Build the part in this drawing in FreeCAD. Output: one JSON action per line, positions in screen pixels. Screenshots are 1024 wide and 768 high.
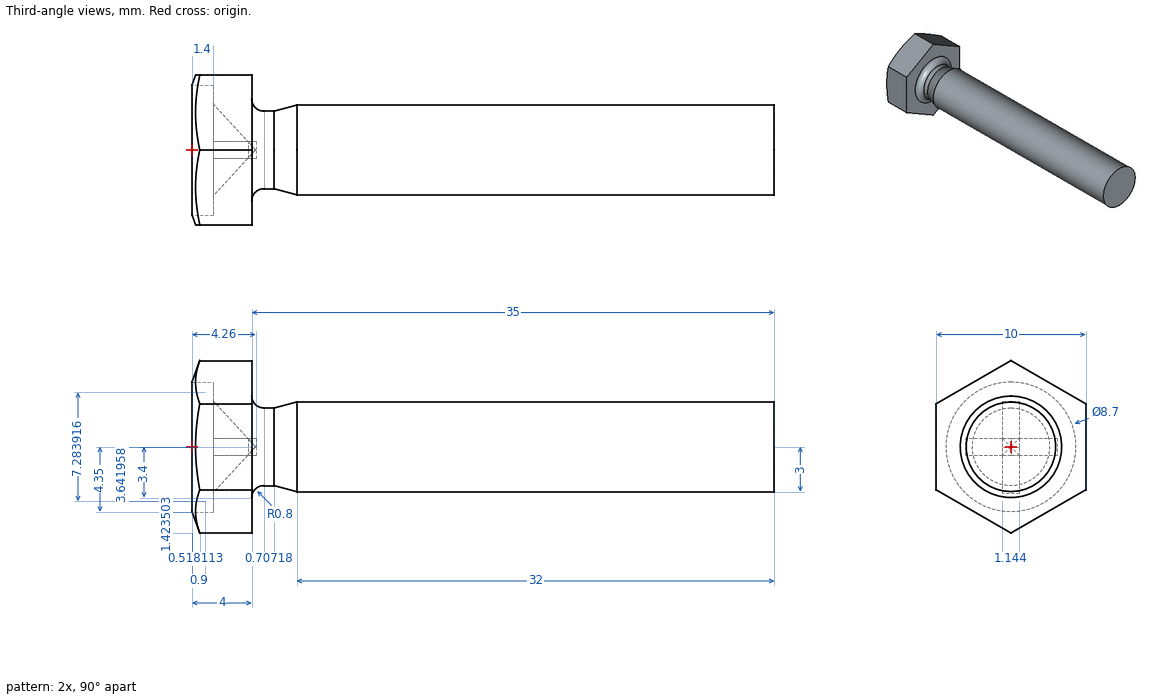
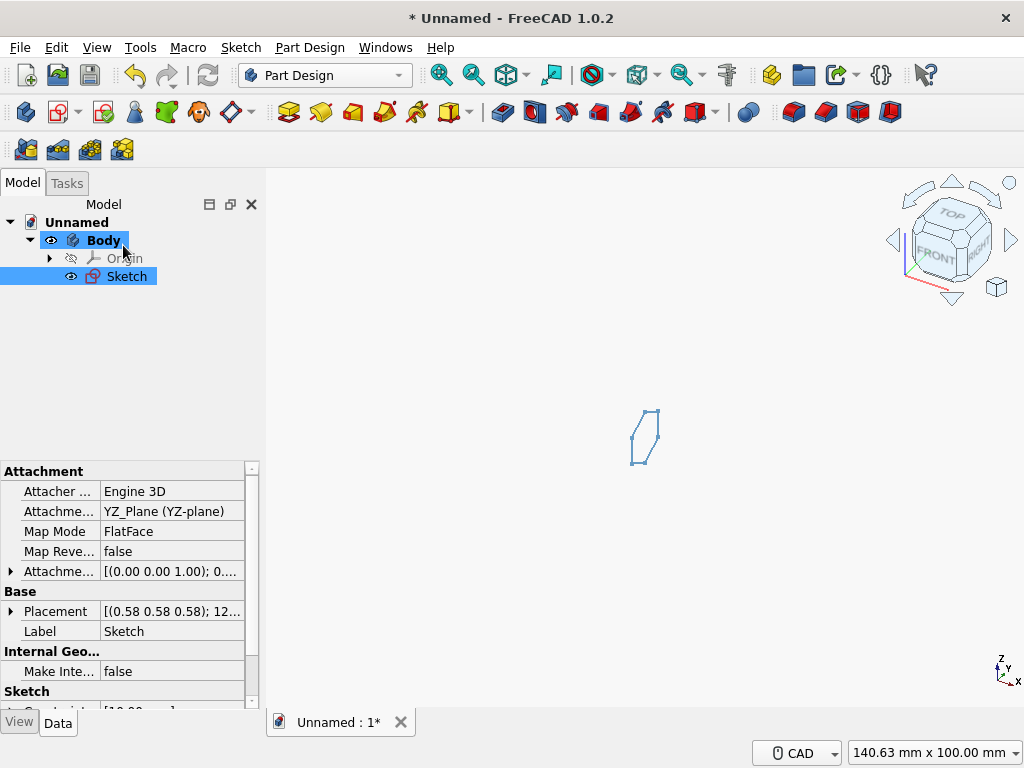
{"action": "left_click", "coordinate": [290, 112]}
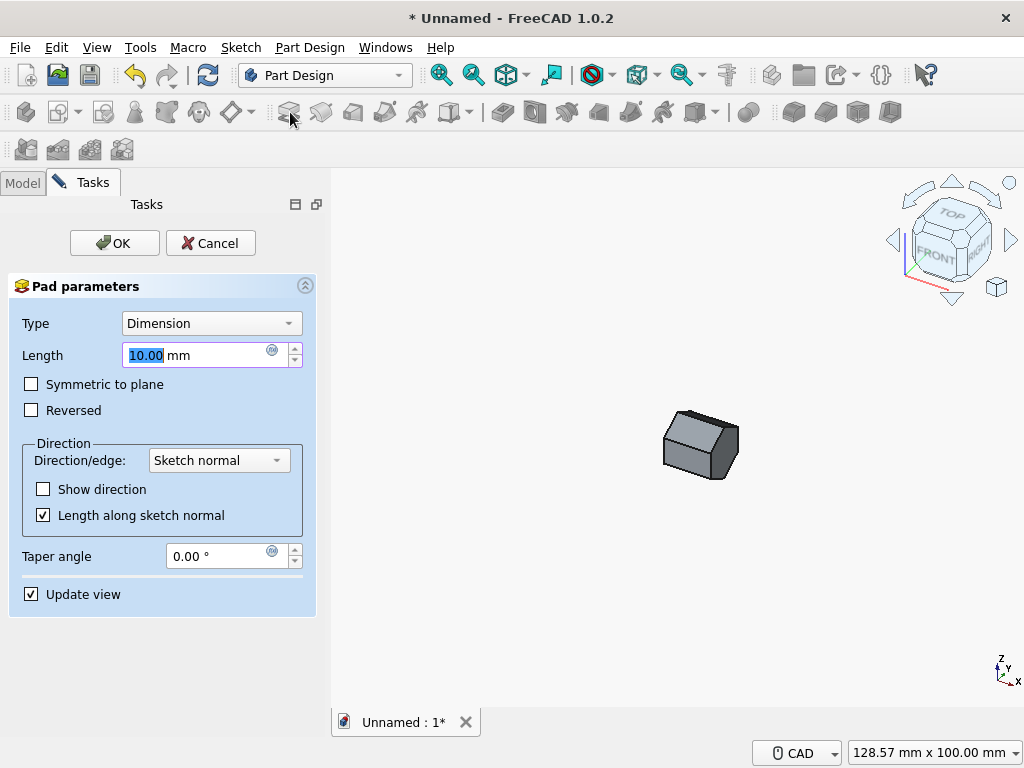
{"action": "type", "text": "4"}
{"action": "key", "text": "Tab"}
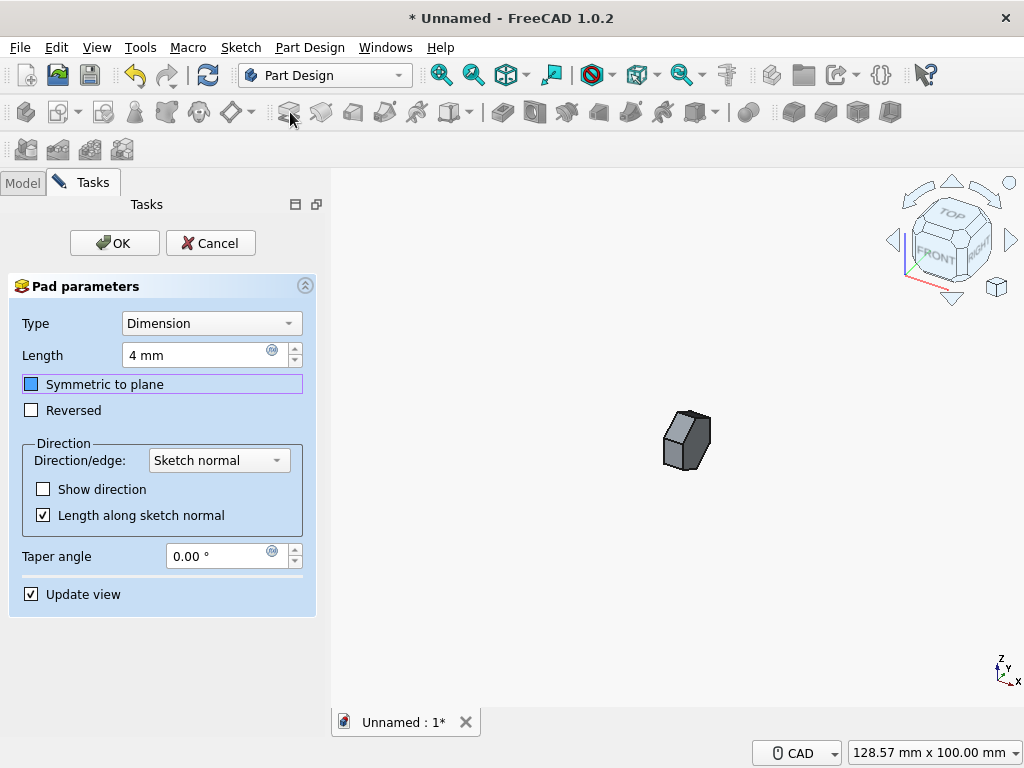
{"action": "left_click", "coordinate": [115, 243]}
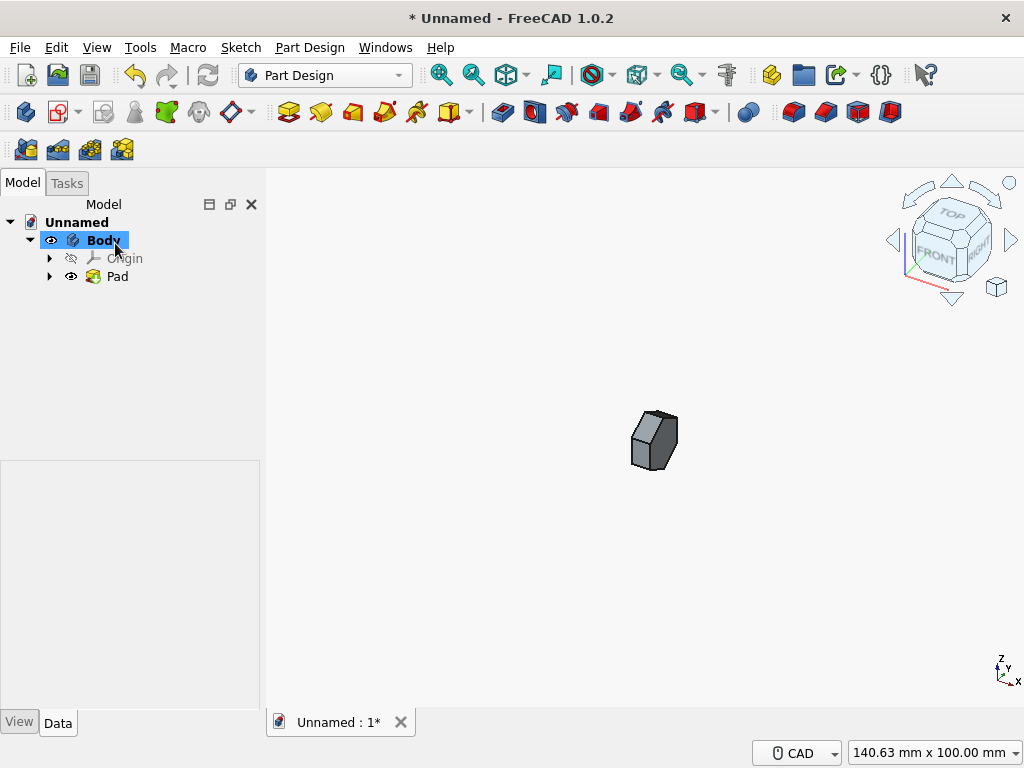
{"action": "left_click", "coordinate": [442, 76]}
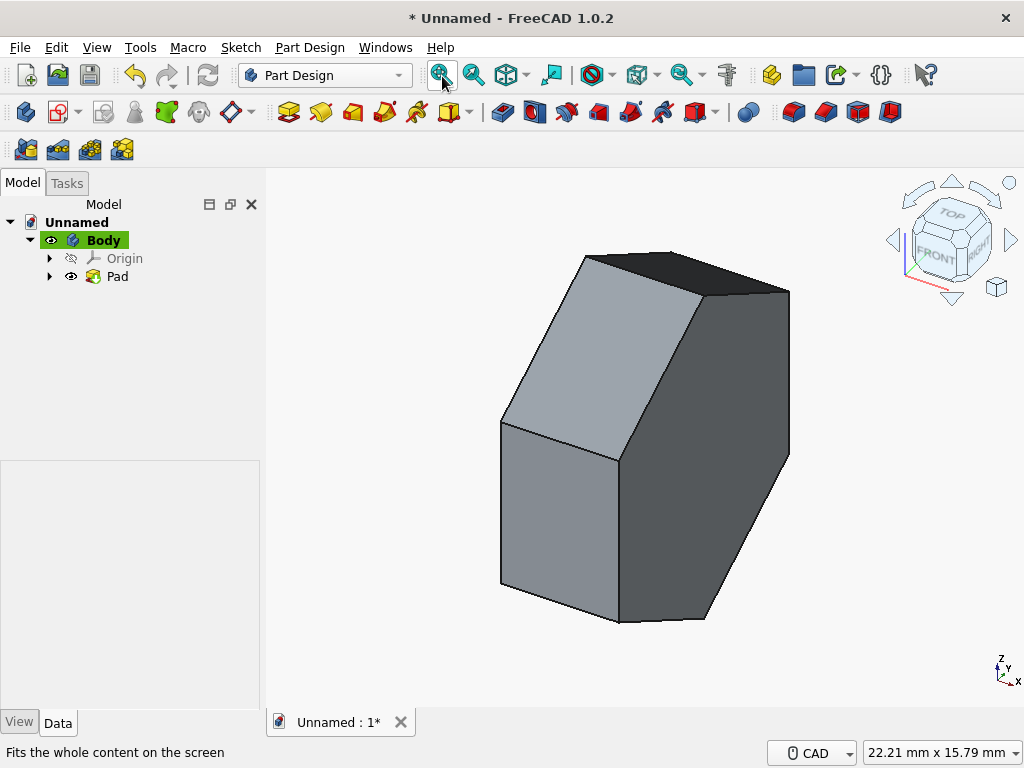
{"action": "left_click", "coordinate": [58, 112]}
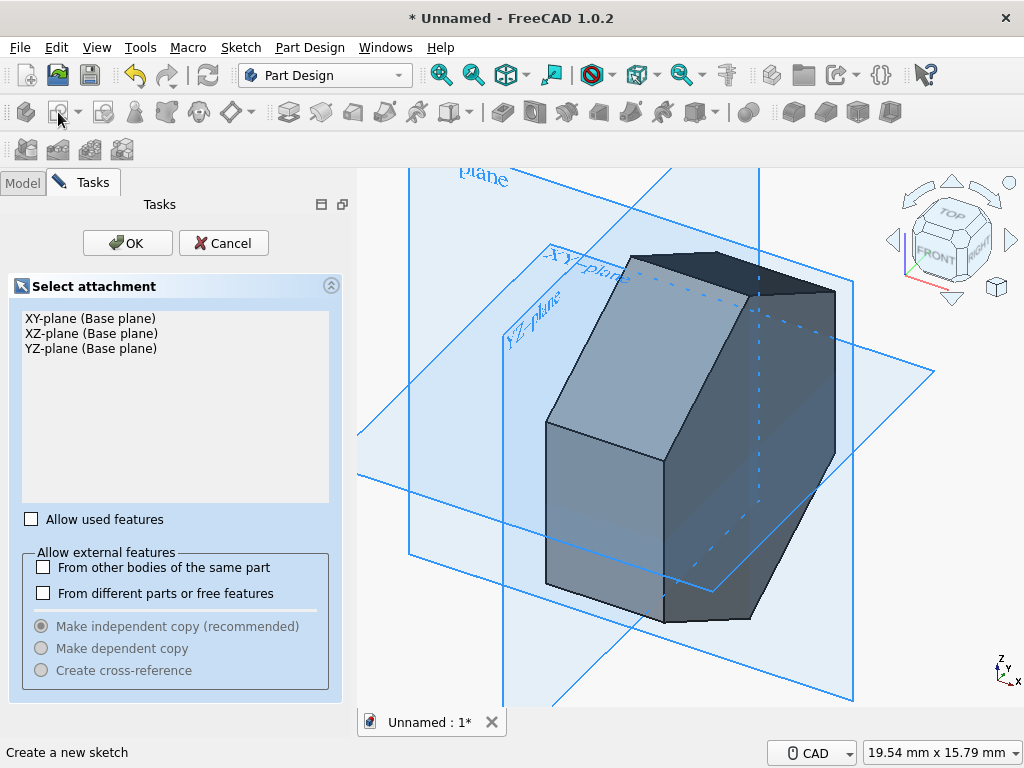
{"action": "left_click", "coordinate": [82, 334]}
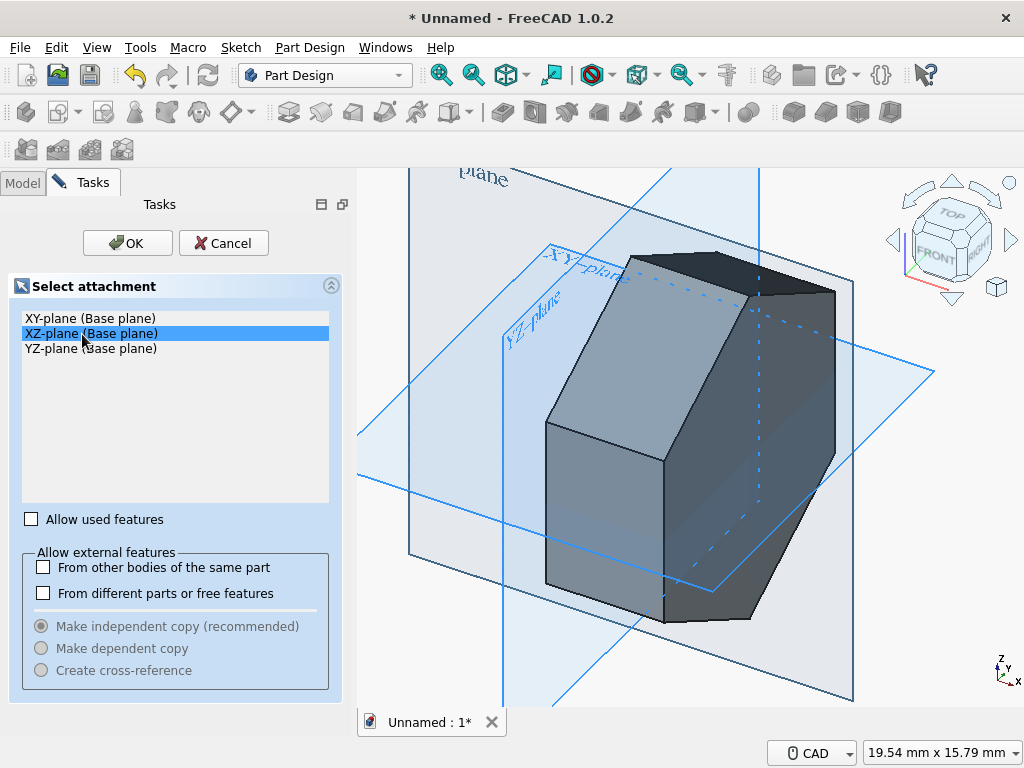
{"action": "left_click", "coordinate": [128, 243]}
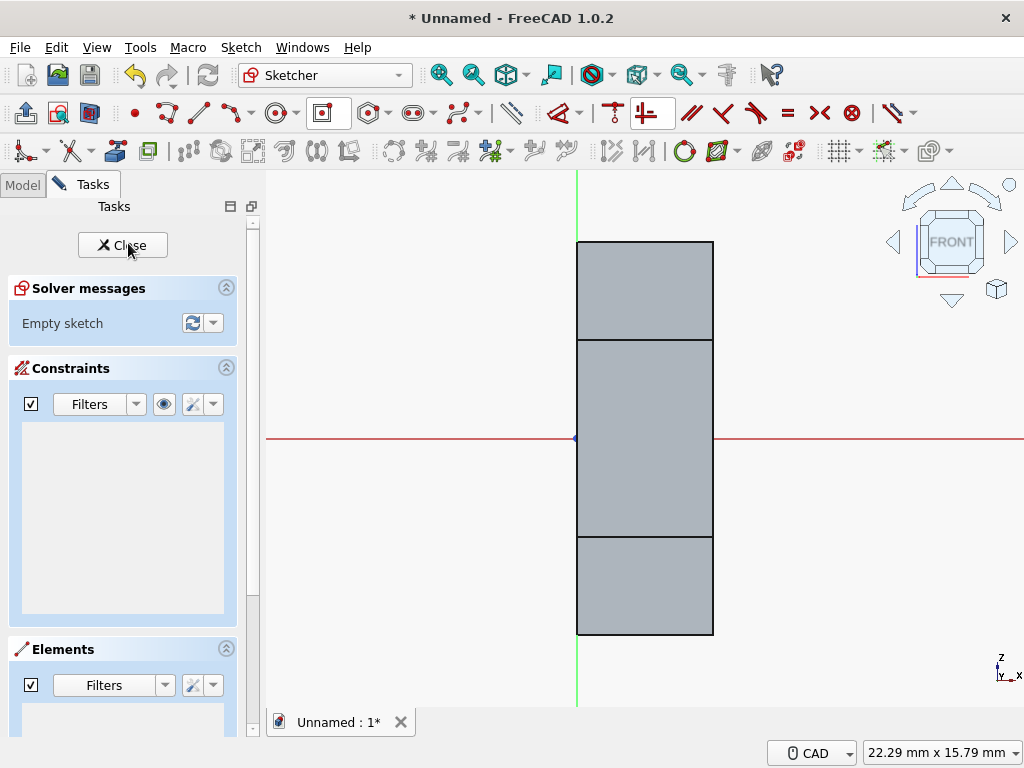
{"action": "left_click", "coordinate": [90, 114]}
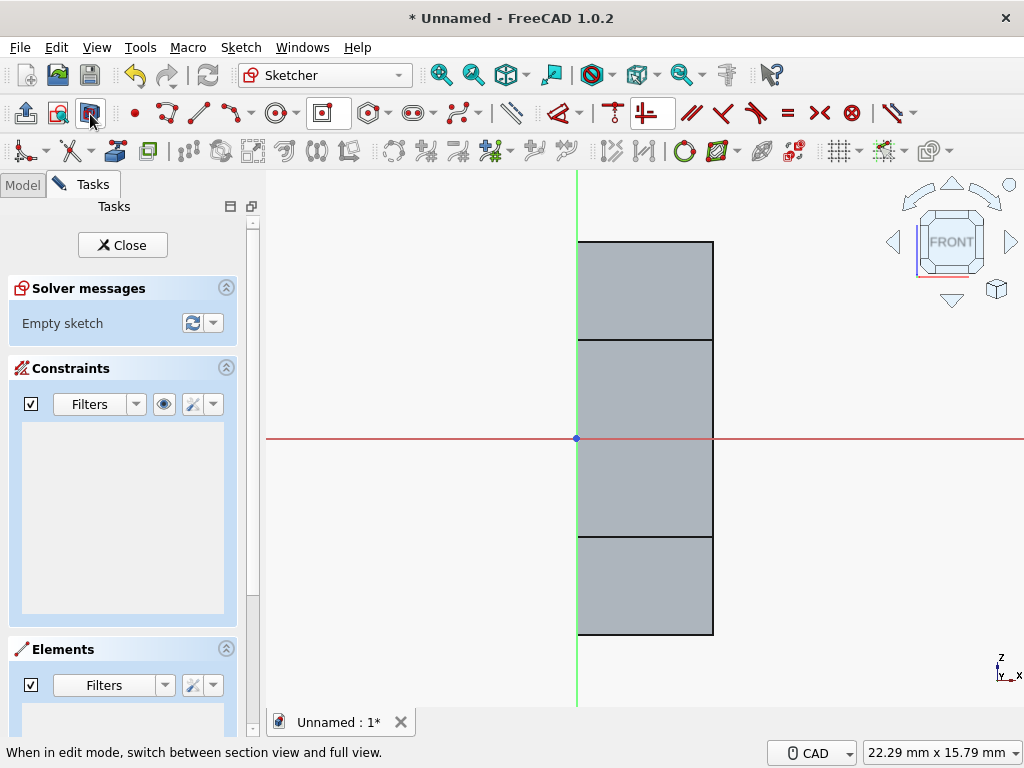
{"action": "scroll", "coordinate": [294, 414], "scroll_direction": "down", "scroll_amount": 6}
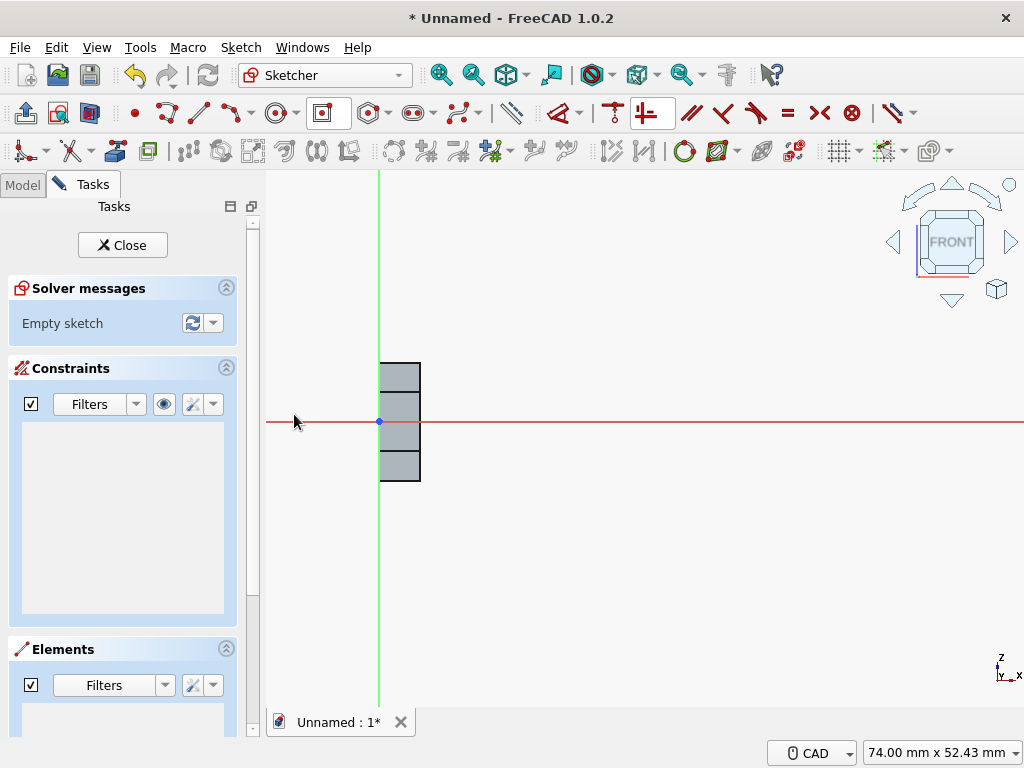
{"action": "left_click", "coordinate": [168, 114]}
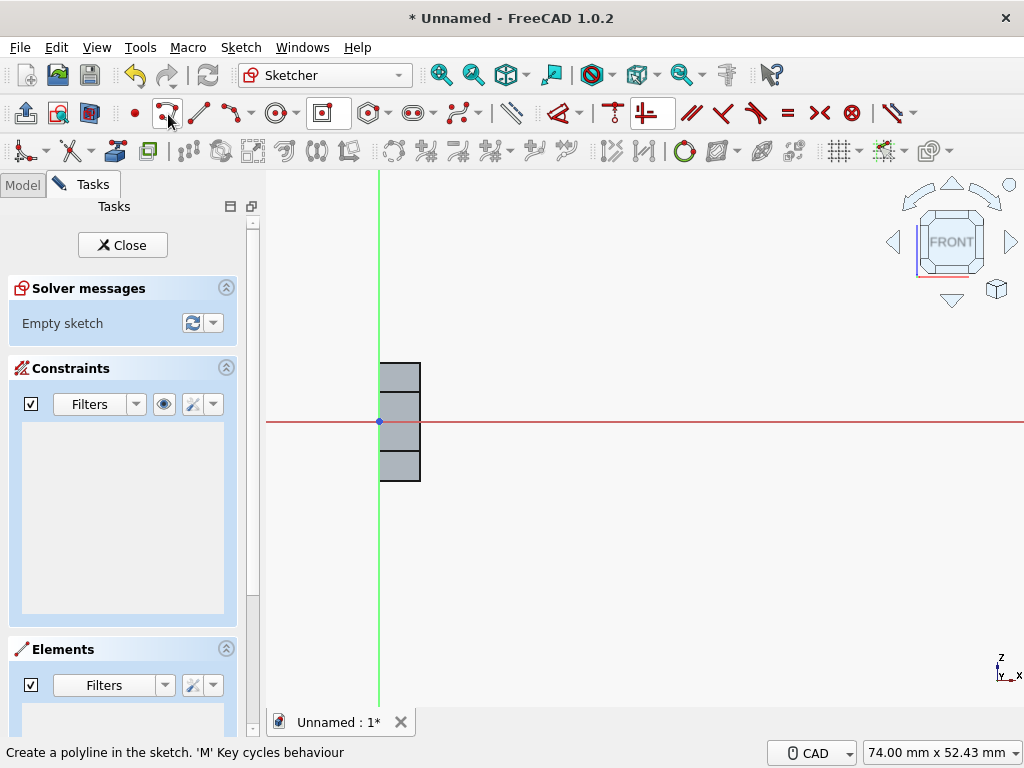
{"action": "left_click", "coordinate": [420, 457]}
{"action": "left_click", "coordinate": [420, 422]}
{"action": "left_click", "coordinate": [779, 431]}
{"action": "left_click", "coordinate": [779, 452]}
{"action": "left_click", "coordinate": [451, 452]}
{"action": "left_click", "coordinate": [436, 448]}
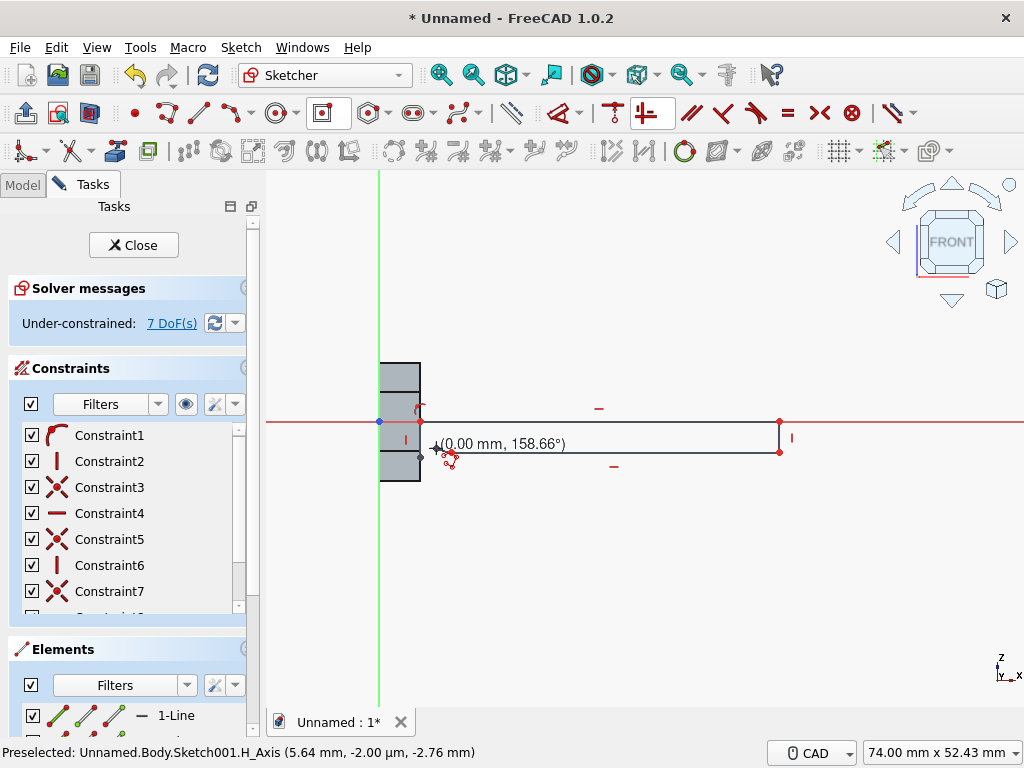
{"action": "scroll", "coordinate": [428, 448], "scroll_direction": "up", "scroll_amount": 4}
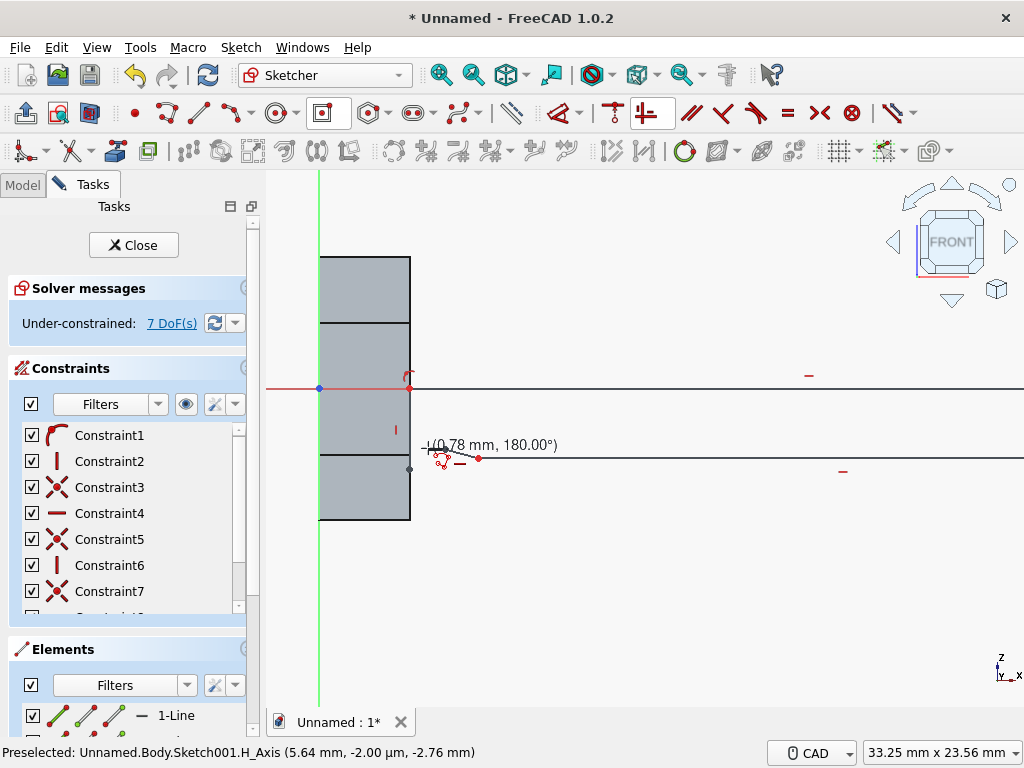
{"action": "left_click", "coordinate": [429, 447]}
{"action": "right_click", "coordinate": [429, 447]}